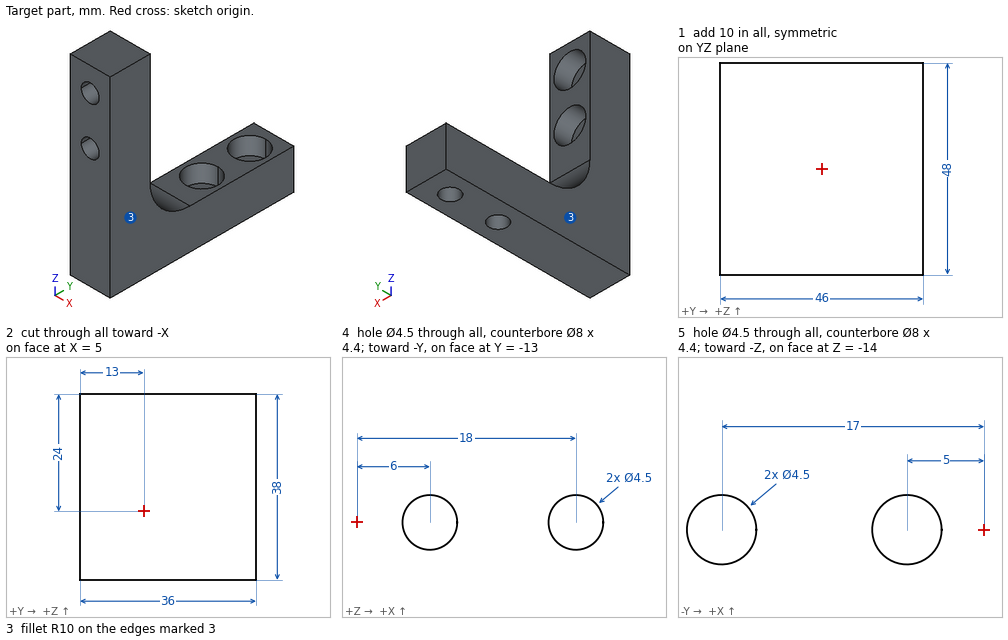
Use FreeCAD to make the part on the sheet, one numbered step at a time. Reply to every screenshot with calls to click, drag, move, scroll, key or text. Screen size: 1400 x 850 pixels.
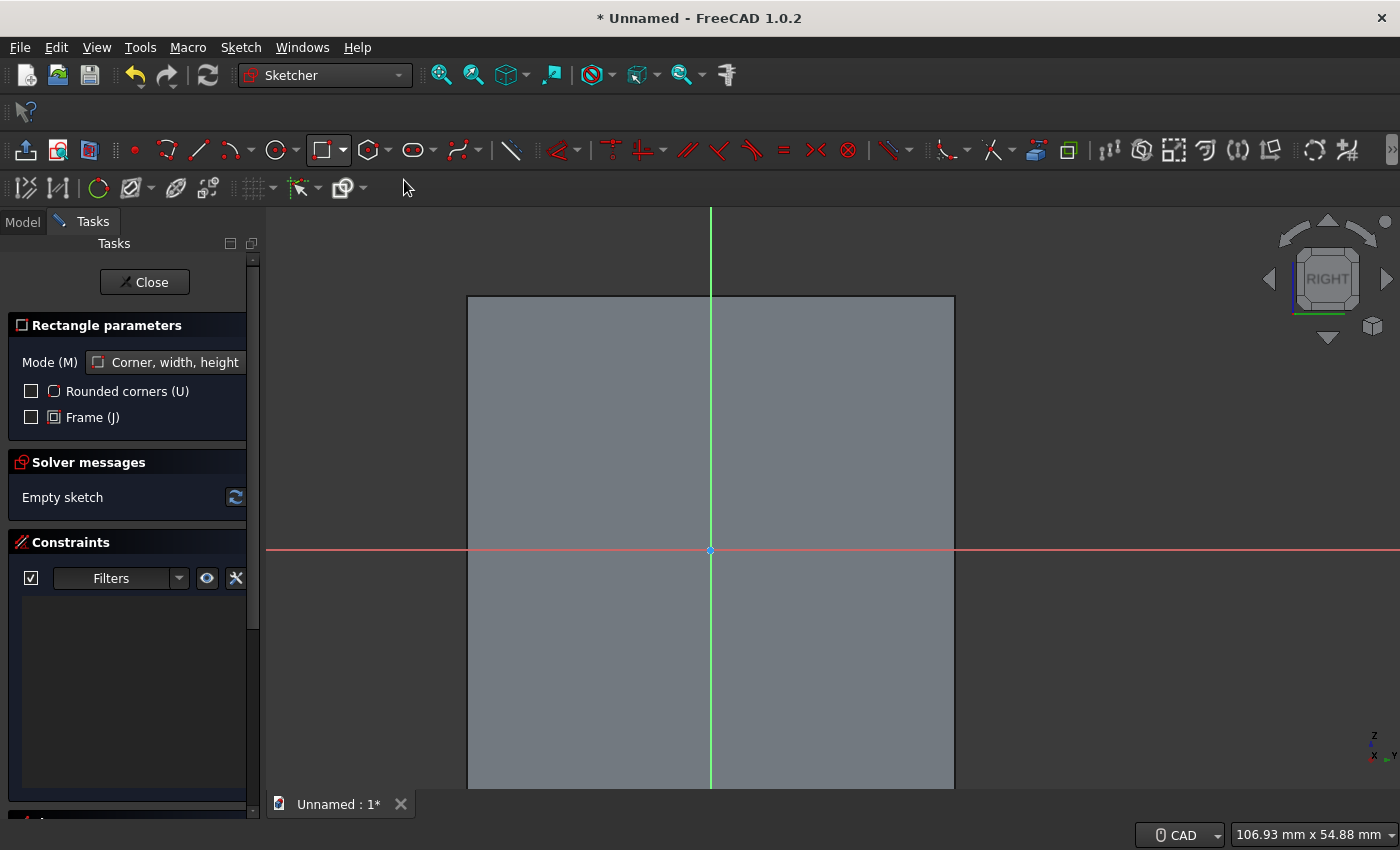
click(573, 296)
move(955, 699)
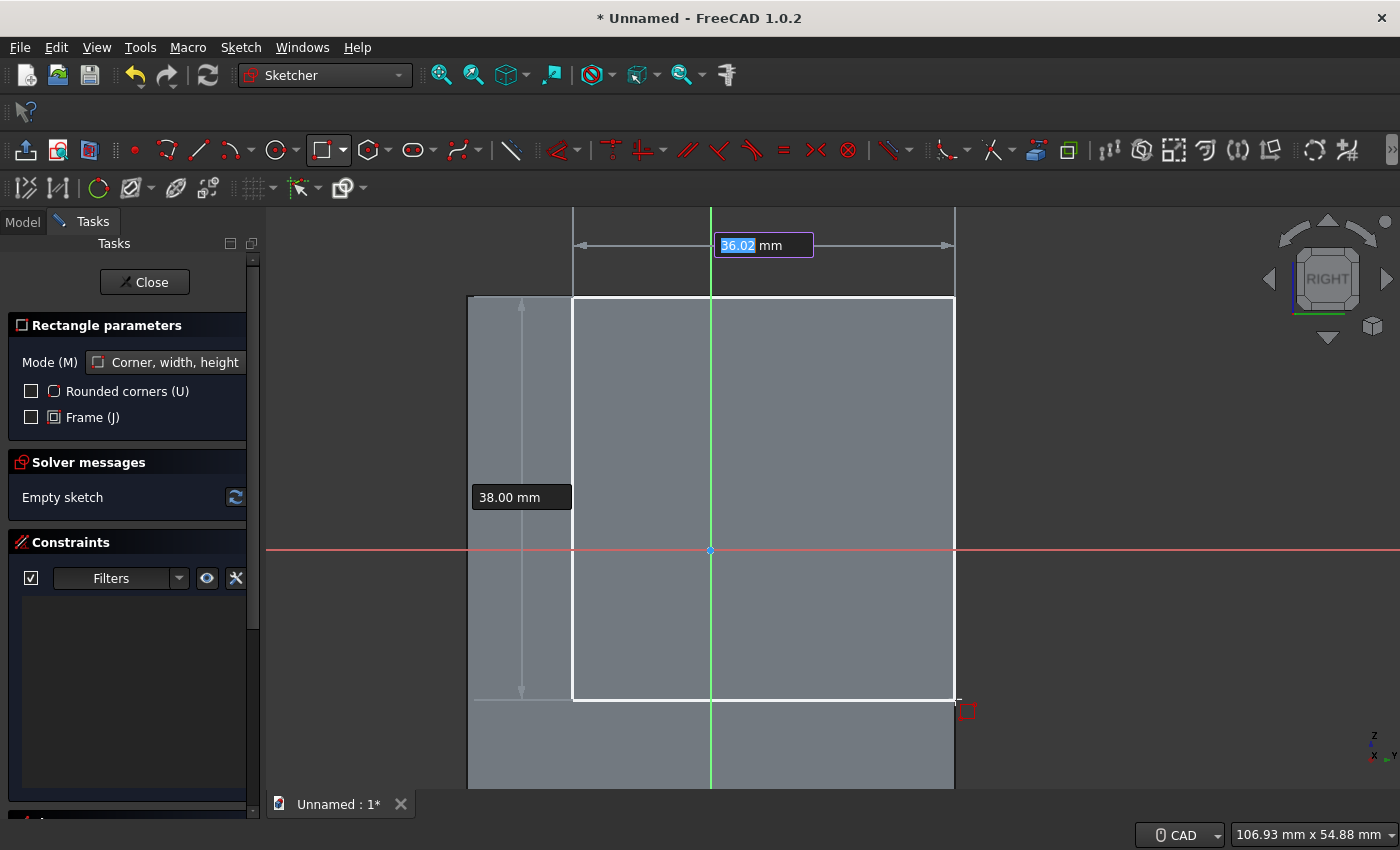
text(36)
key(Tab)
text(38)
key(Return)
key(Escape)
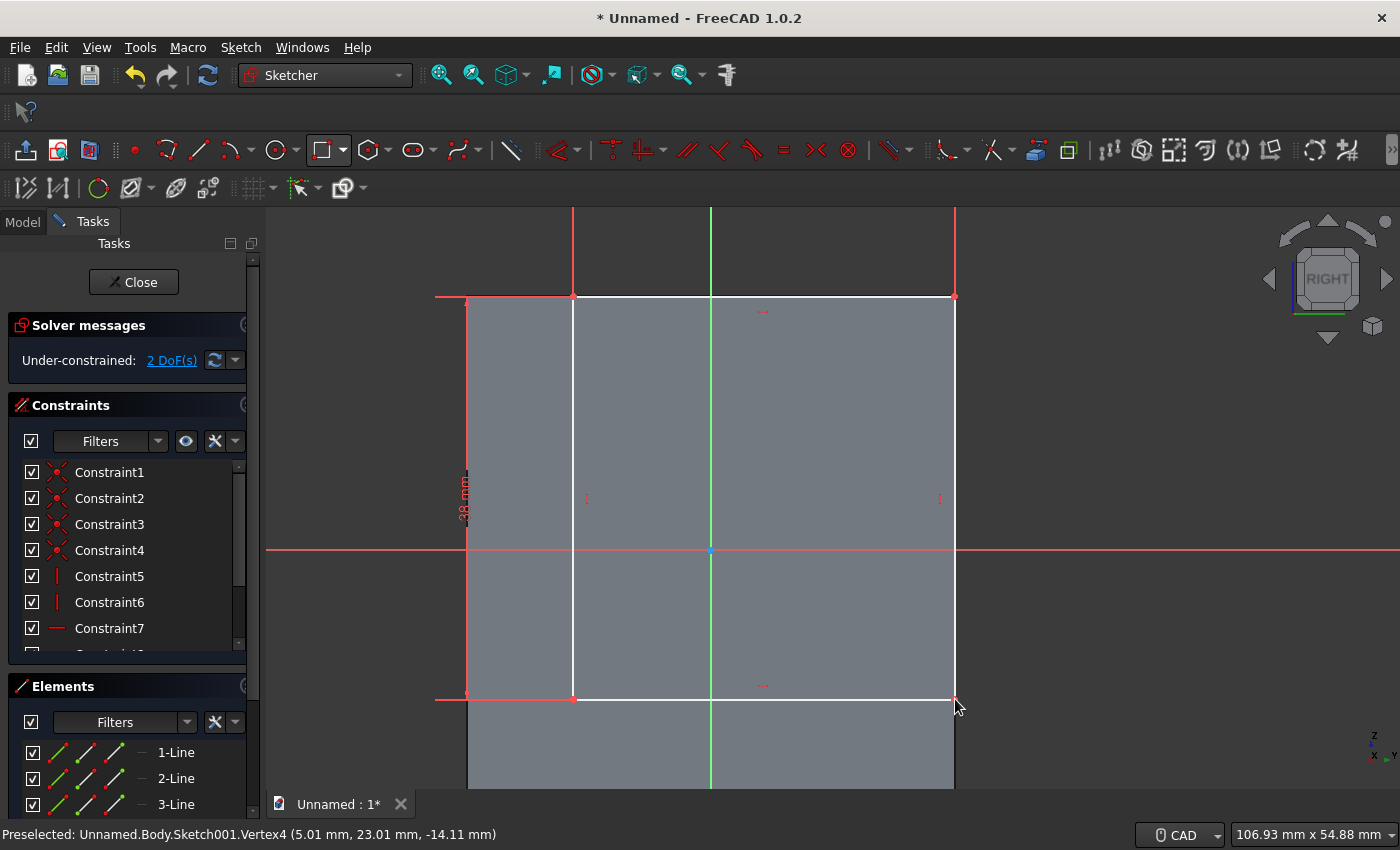
click(558, 150)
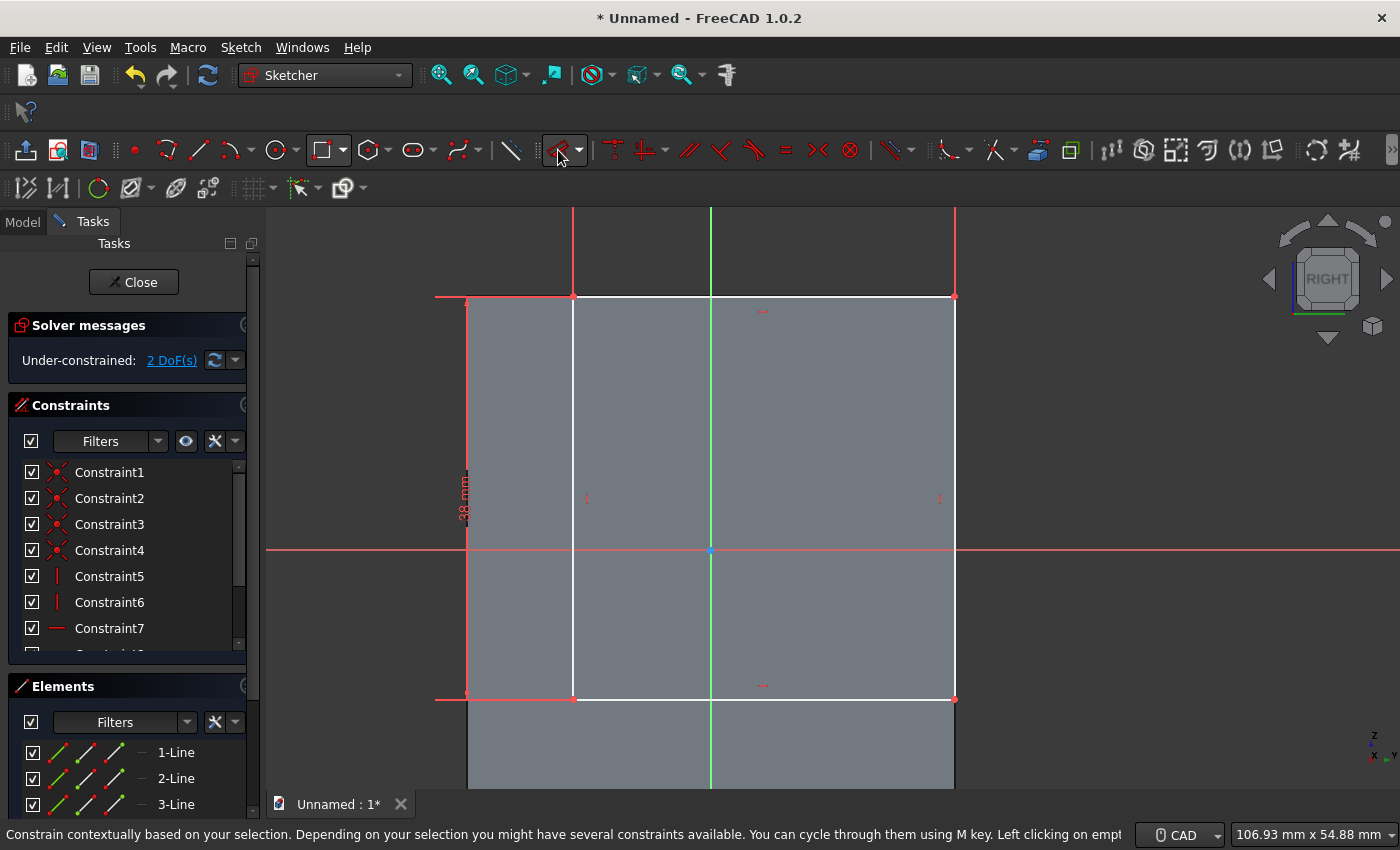
click(573, 297)
click(642, 263)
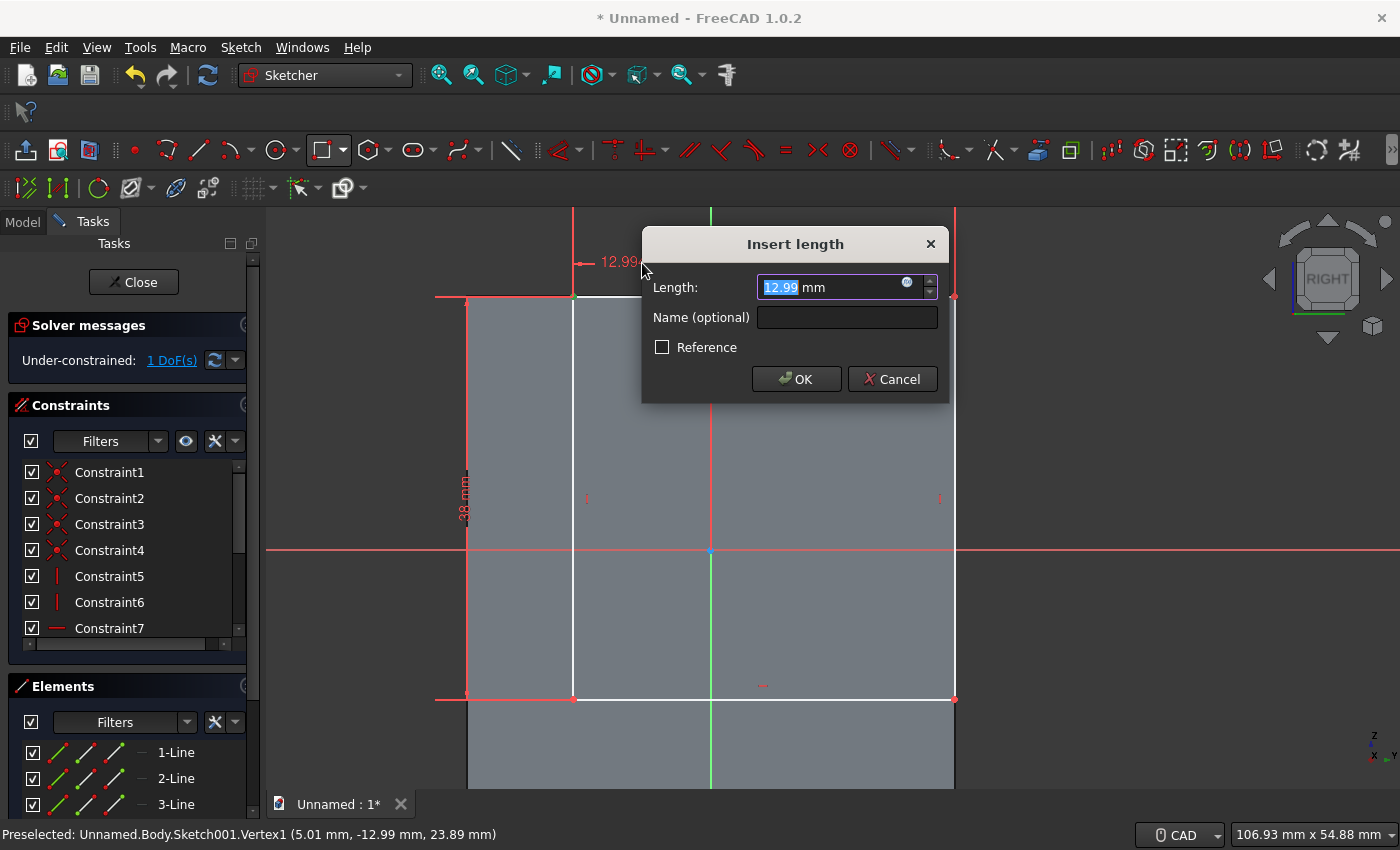
text(13)
key(Return)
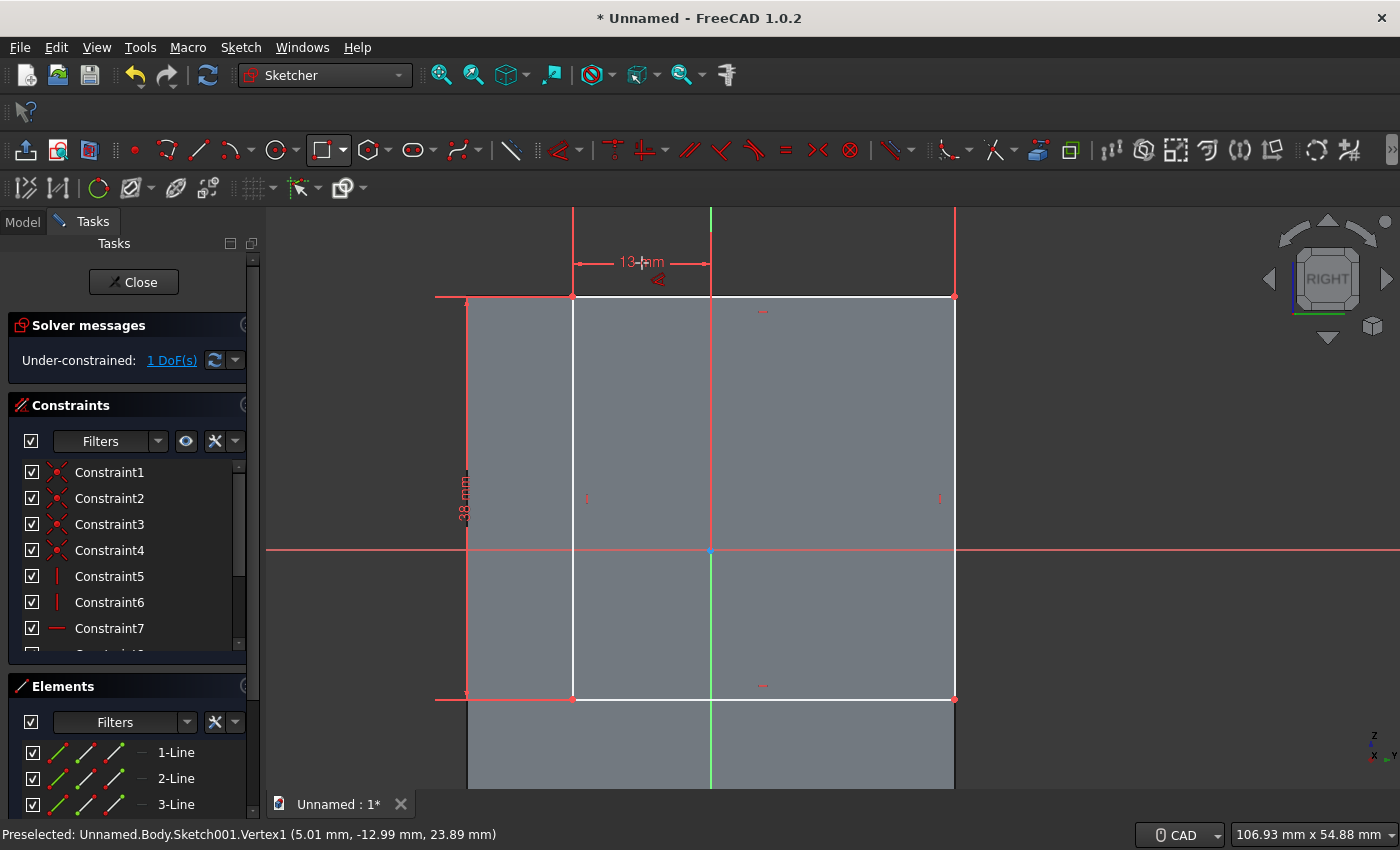
click(573, 297)
click(539, 424)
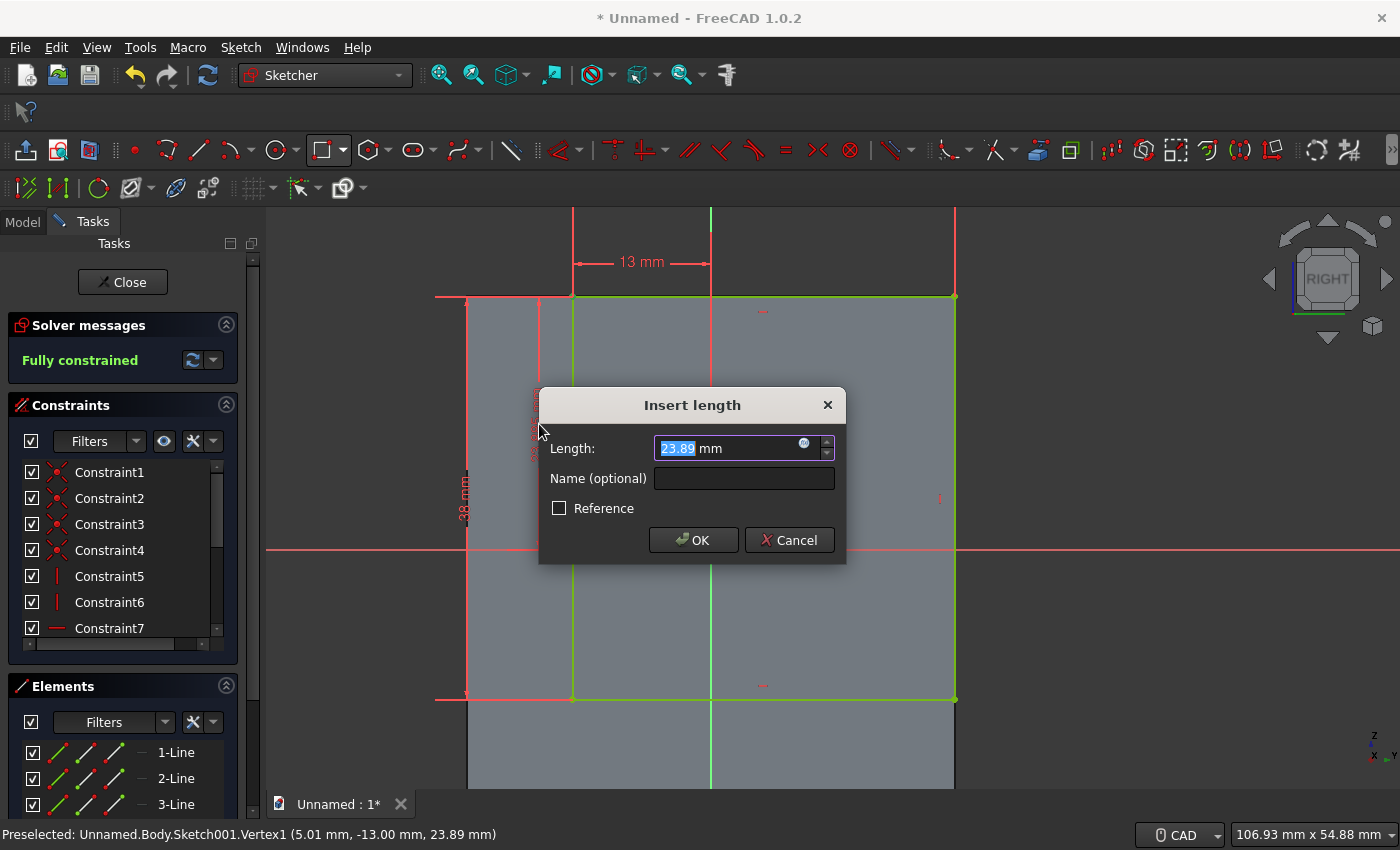
text(24)
key(Return)
key(Escape)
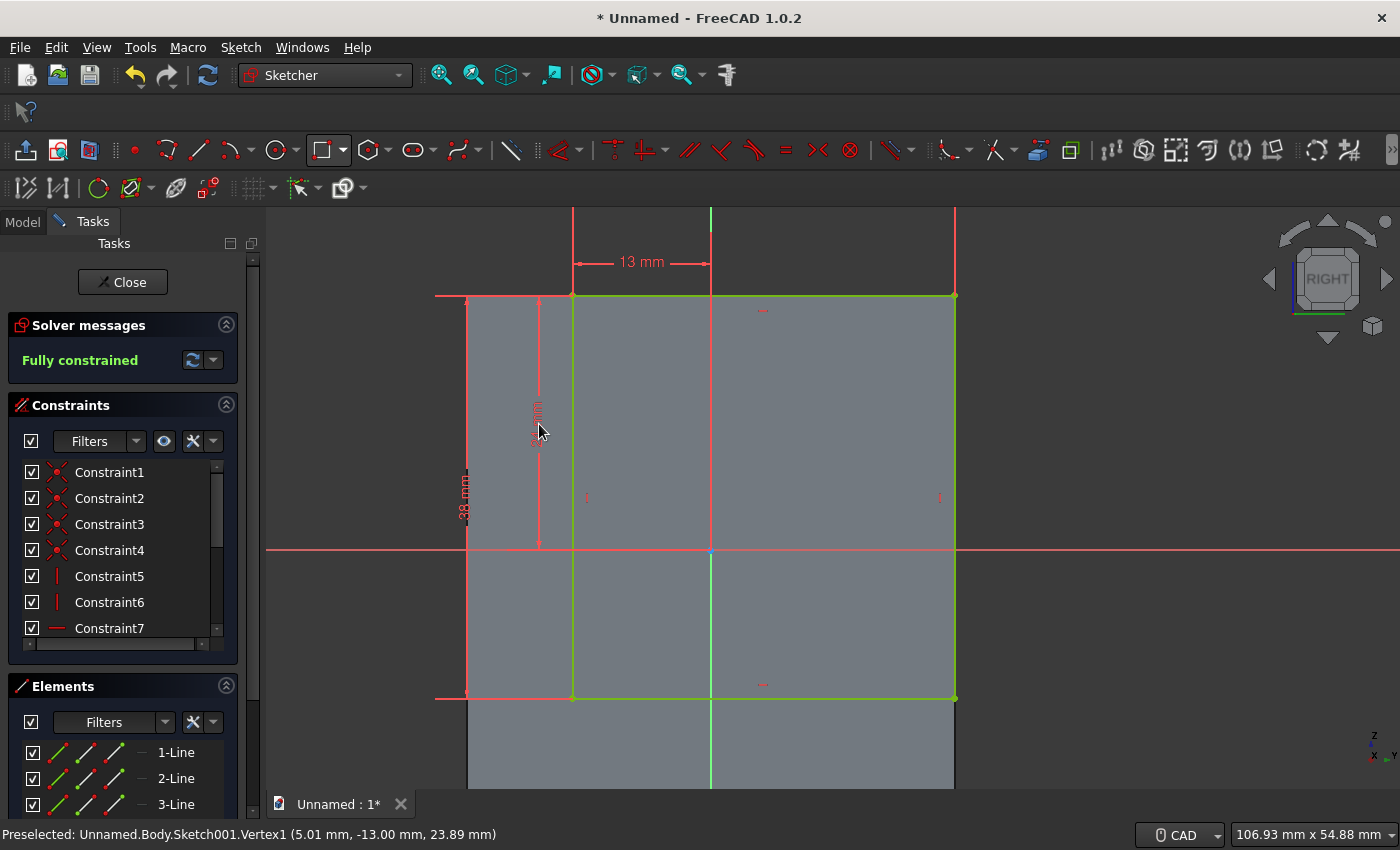
click(123, 282)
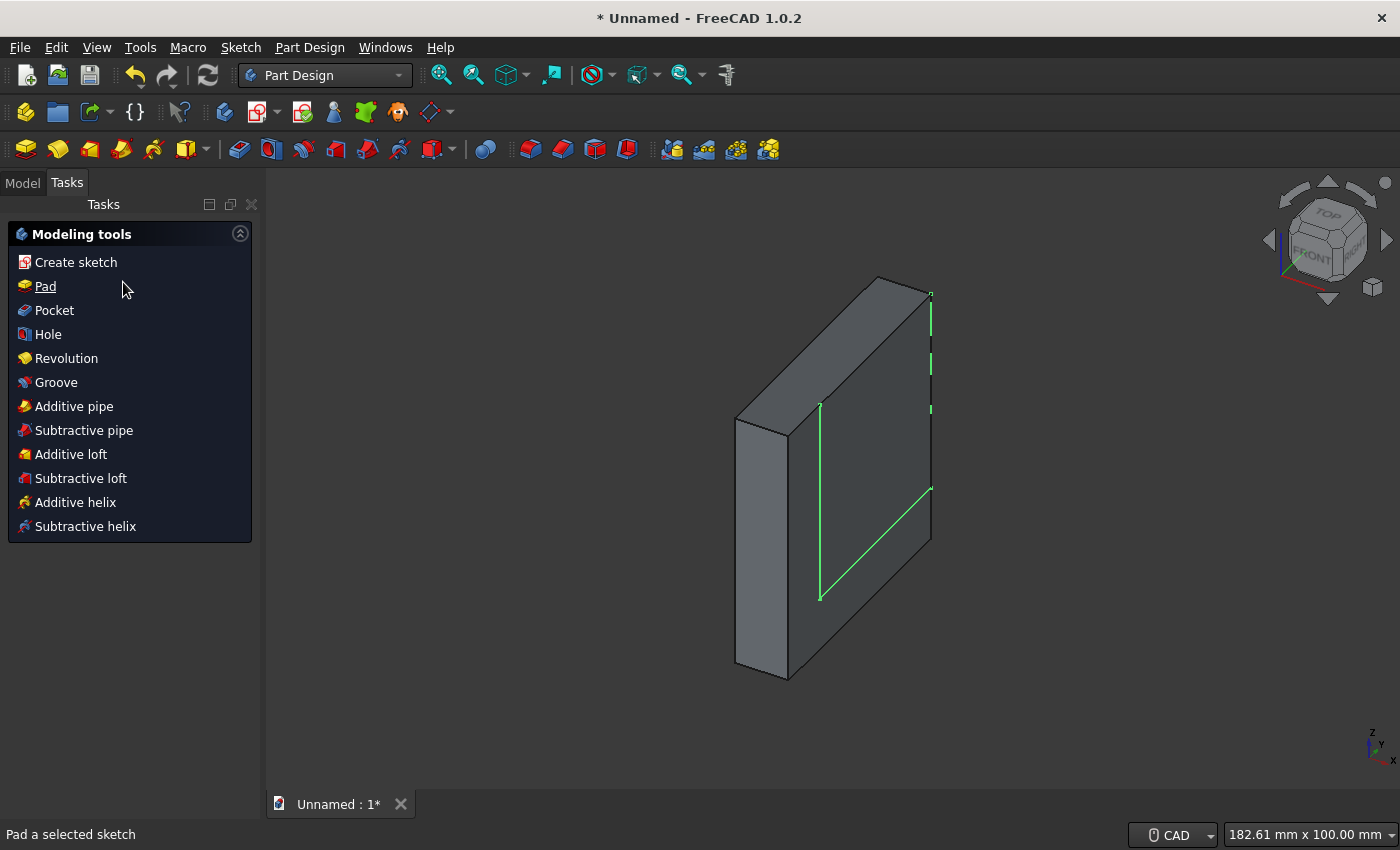
click(240, 150)